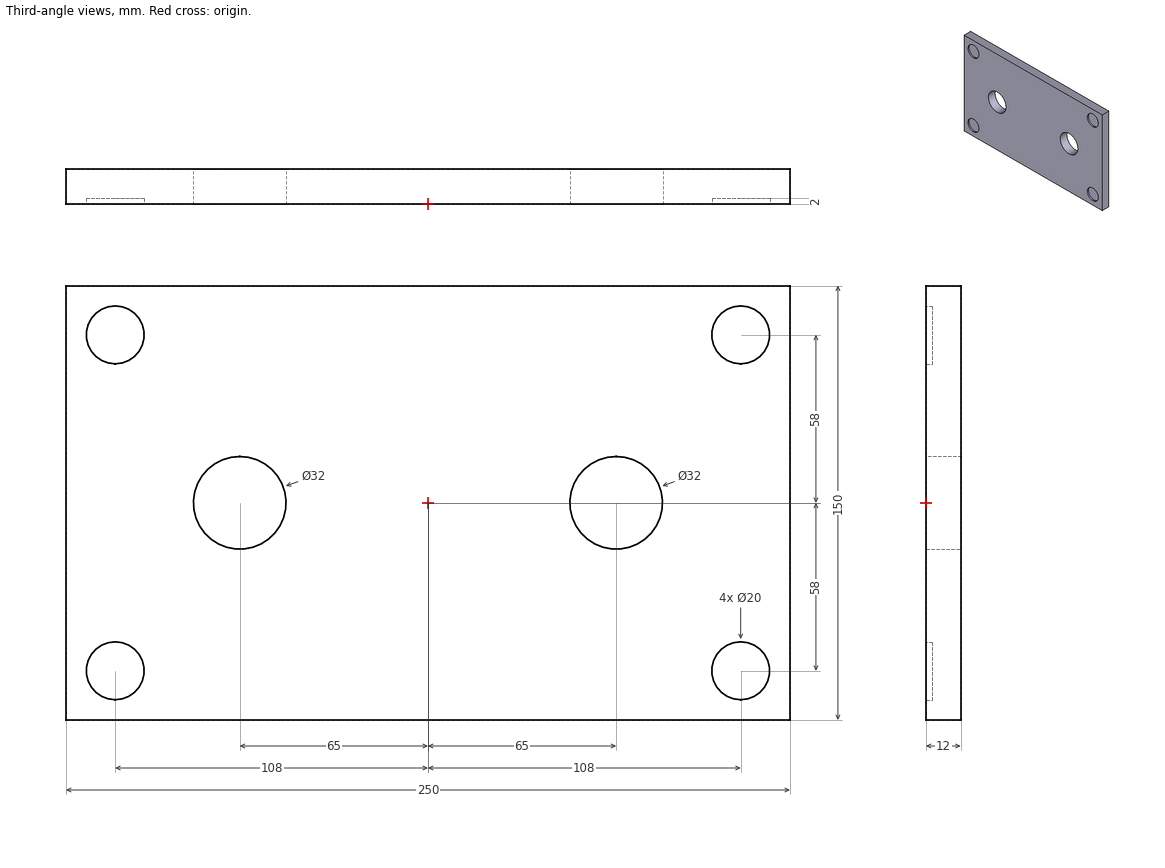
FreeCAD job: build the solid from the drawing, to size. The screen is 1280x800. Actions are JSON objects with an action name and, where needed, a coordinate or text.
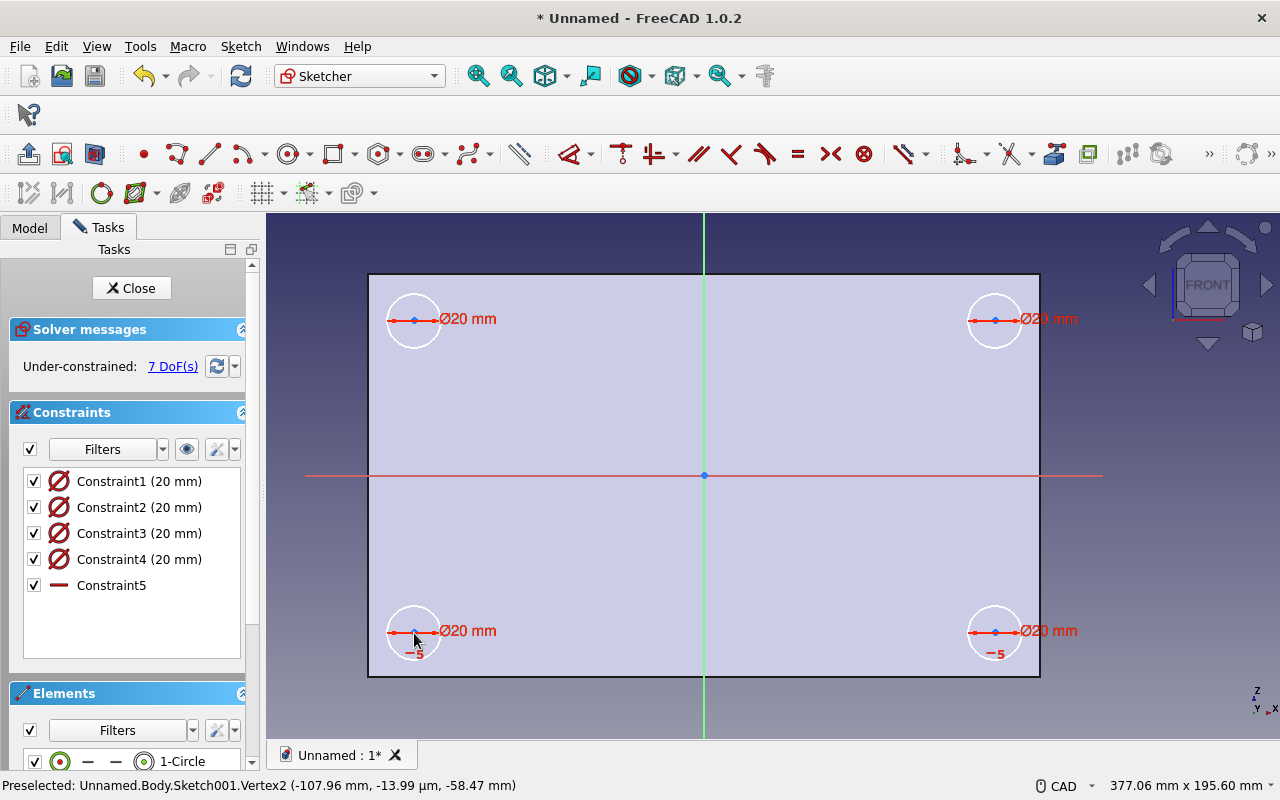
{"action": "left_click", "coordinate": [995, 633]}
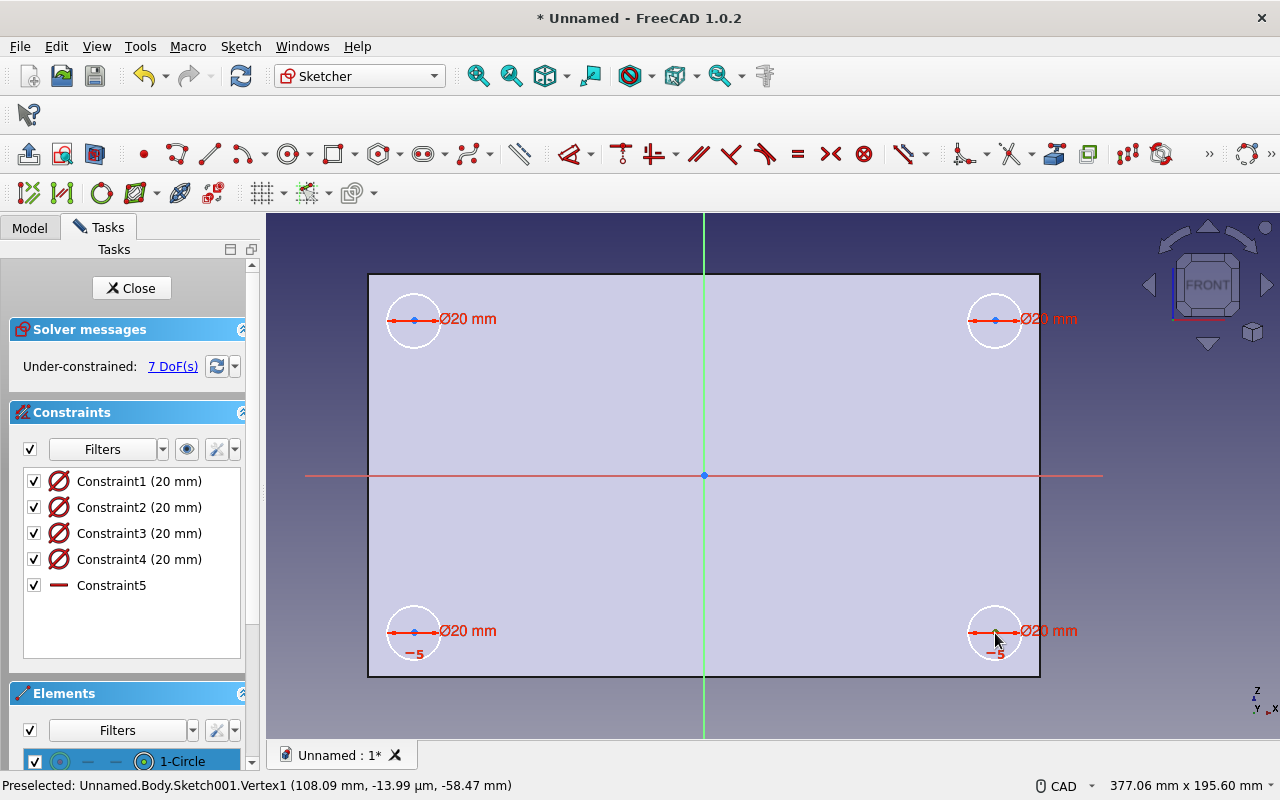
{"action": "left_click", "coordinate": [995, 321]}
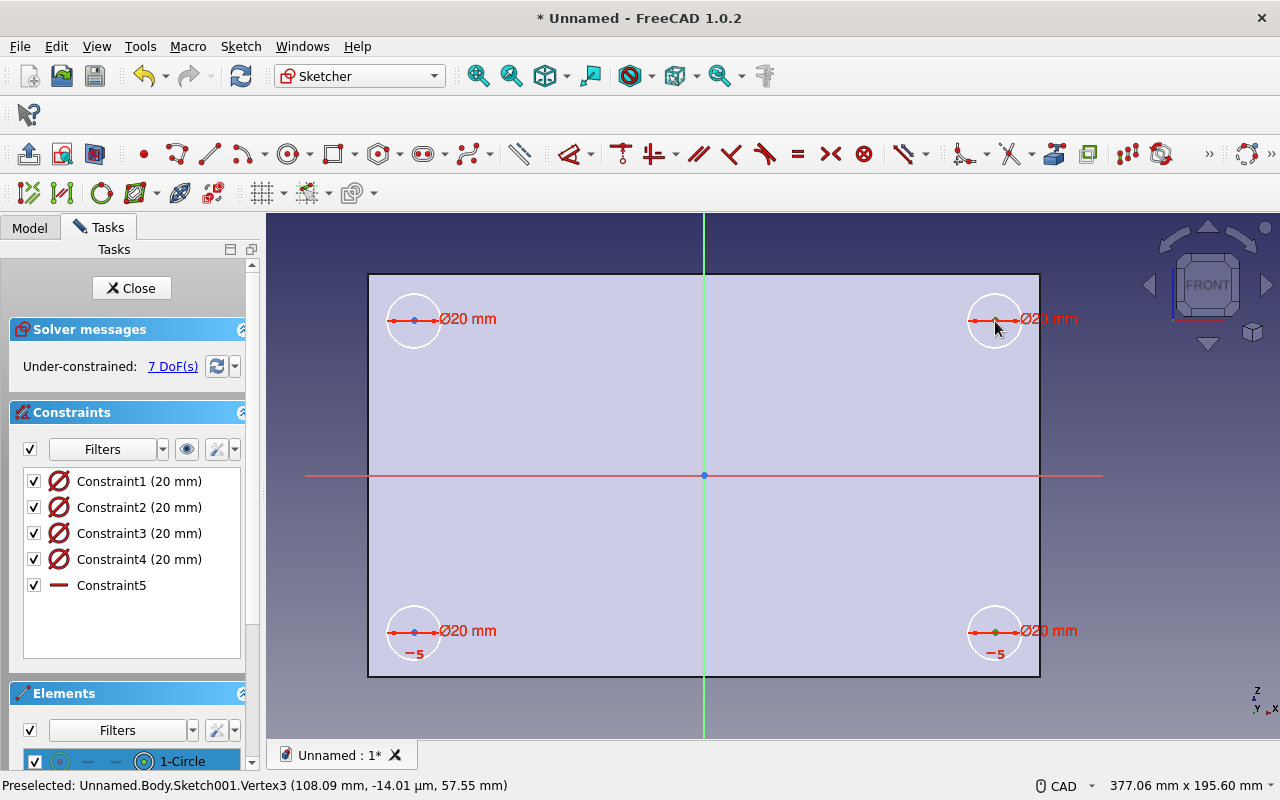
{"action": "left_click", "coordinate": [676, 154]}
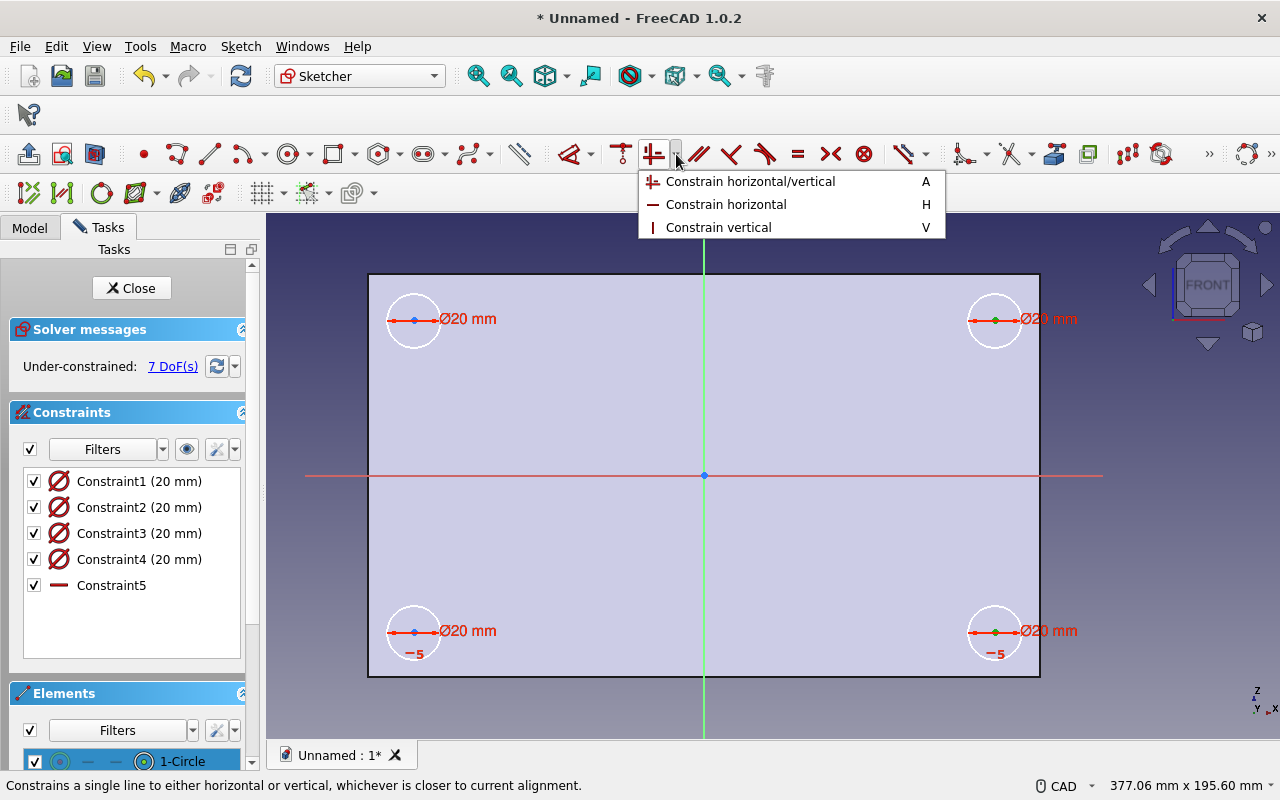
{"action": "left_click", "coordinate": [792, 228]}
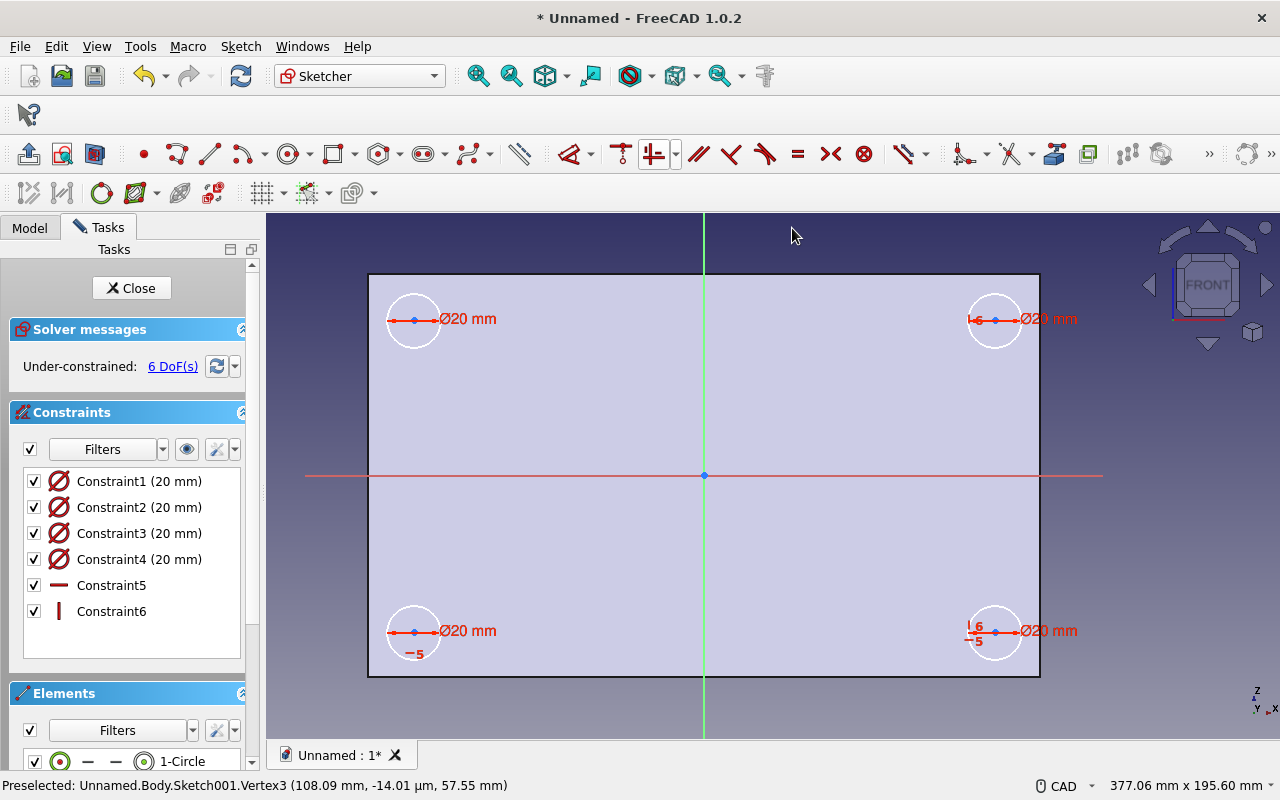
{"action": "left_click", "coordinate": [414, 633]}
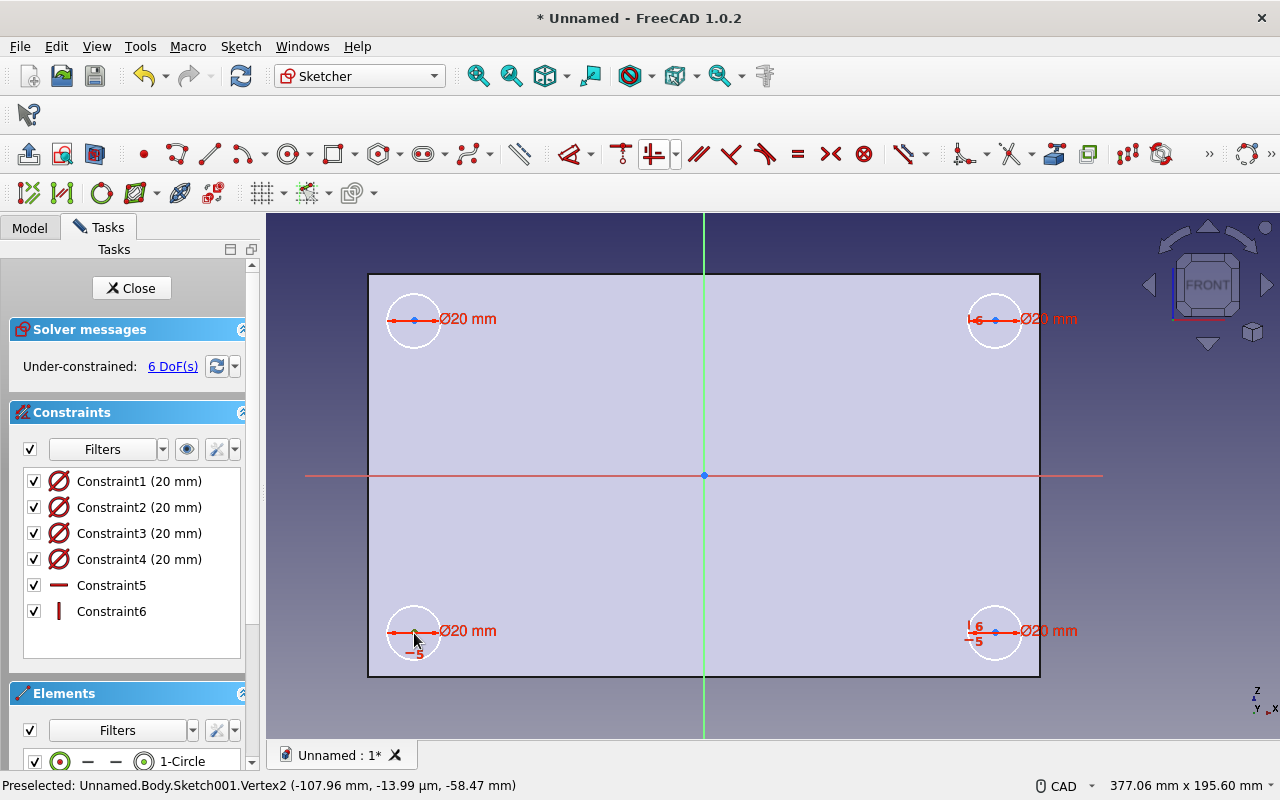
{"action": "left_click", "coordinate": [414, 321]}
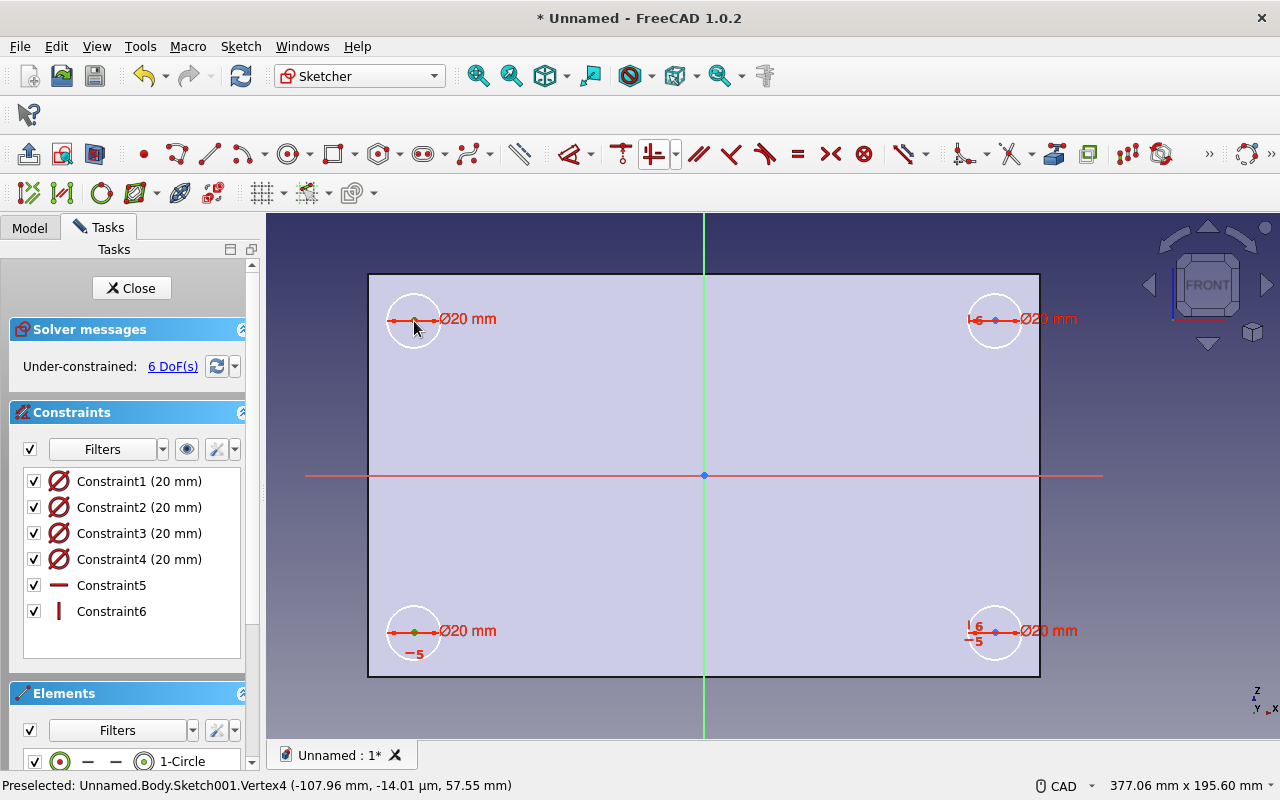
{"action": "left_click", "coordinate": [676, 154]}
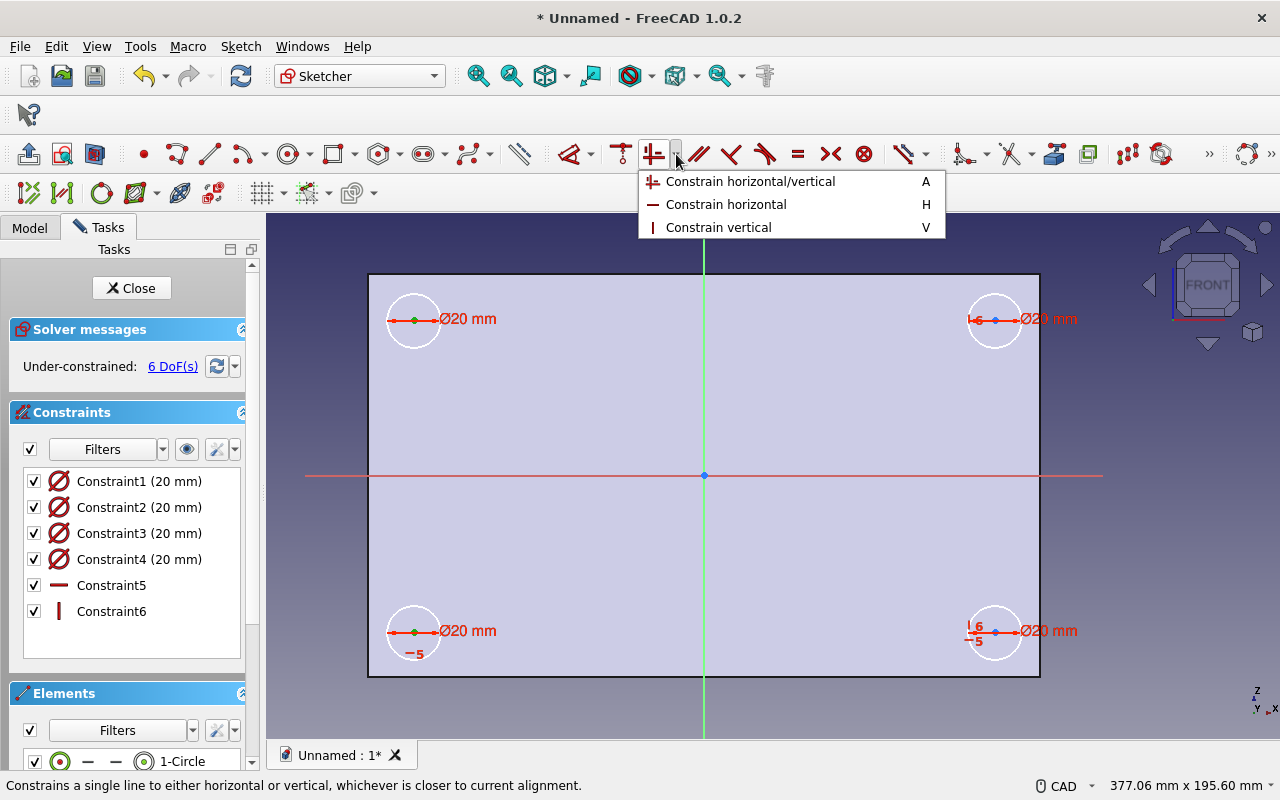
{"action": "left_click", "coordinate": [792, 228]}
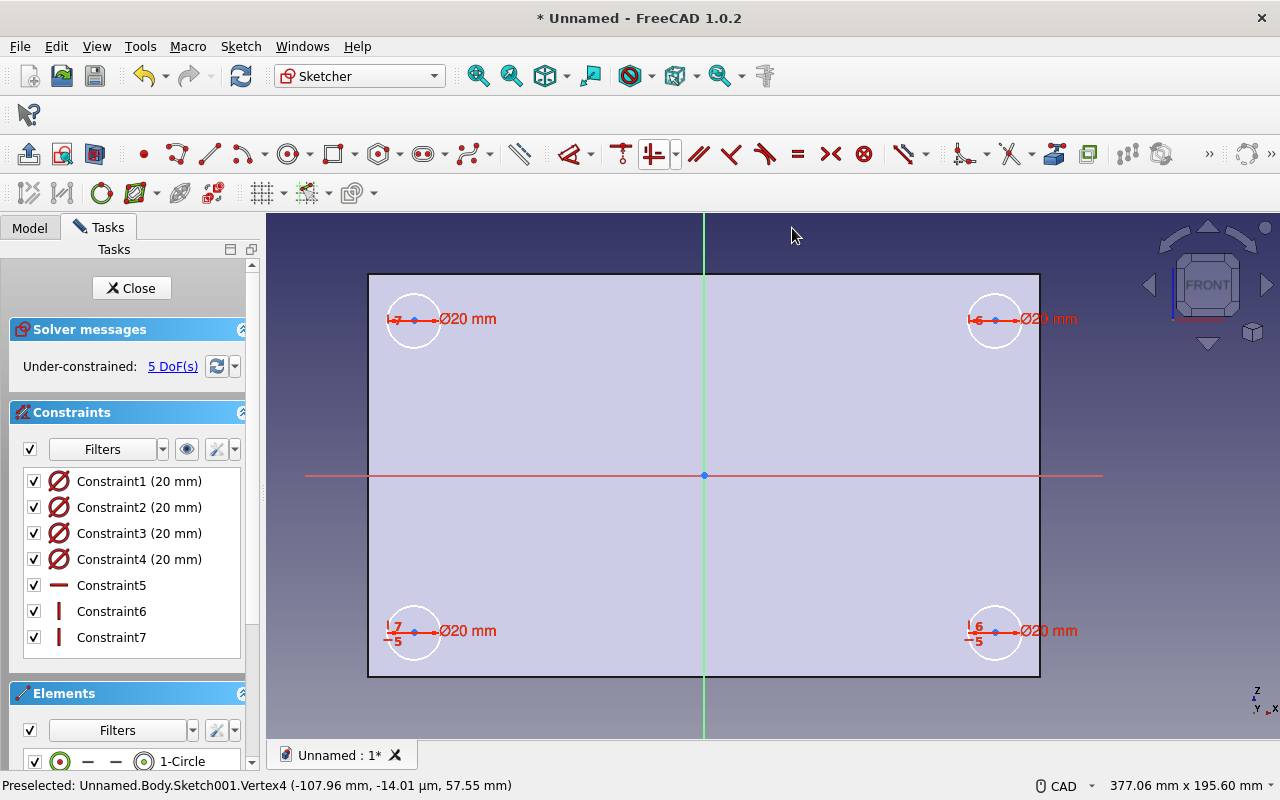
{"action": "left_click", "coordinate": [995, 321]}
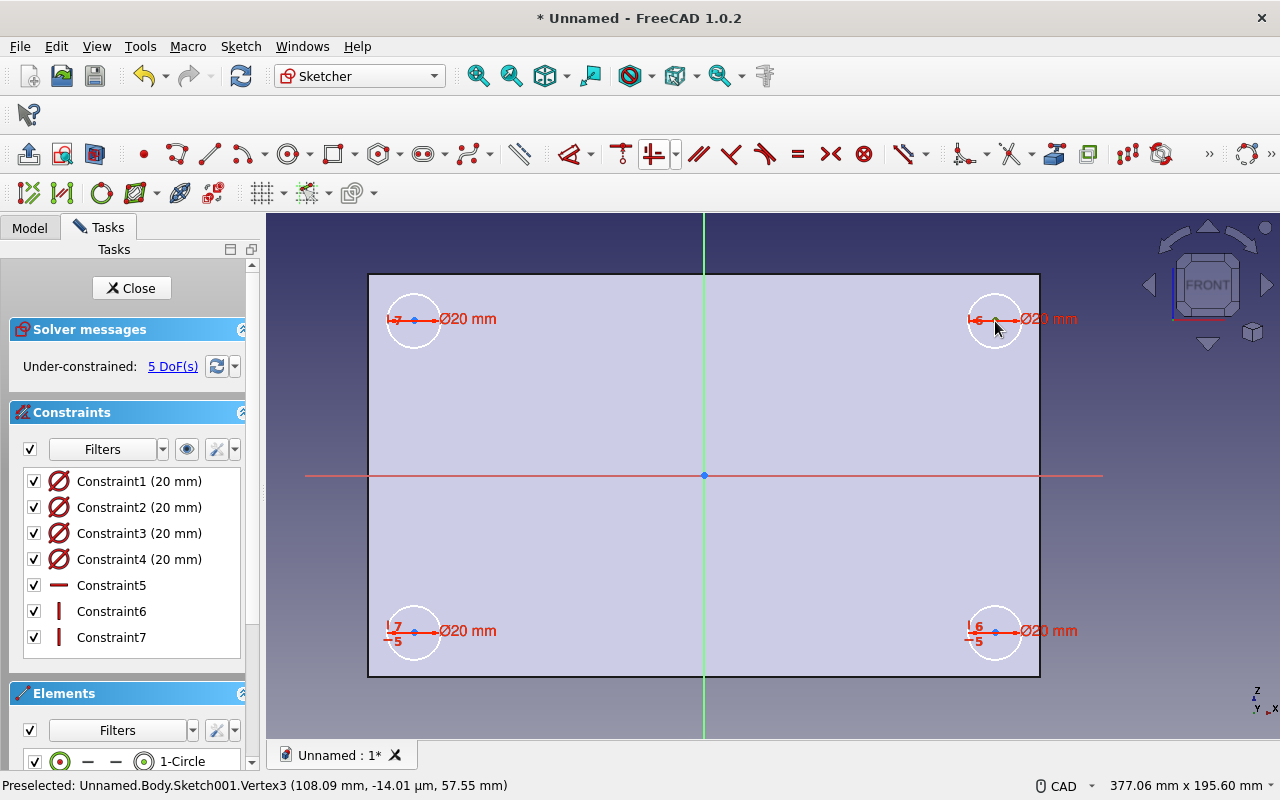
{"action": "left_click", "coordinate": [414, 321]}